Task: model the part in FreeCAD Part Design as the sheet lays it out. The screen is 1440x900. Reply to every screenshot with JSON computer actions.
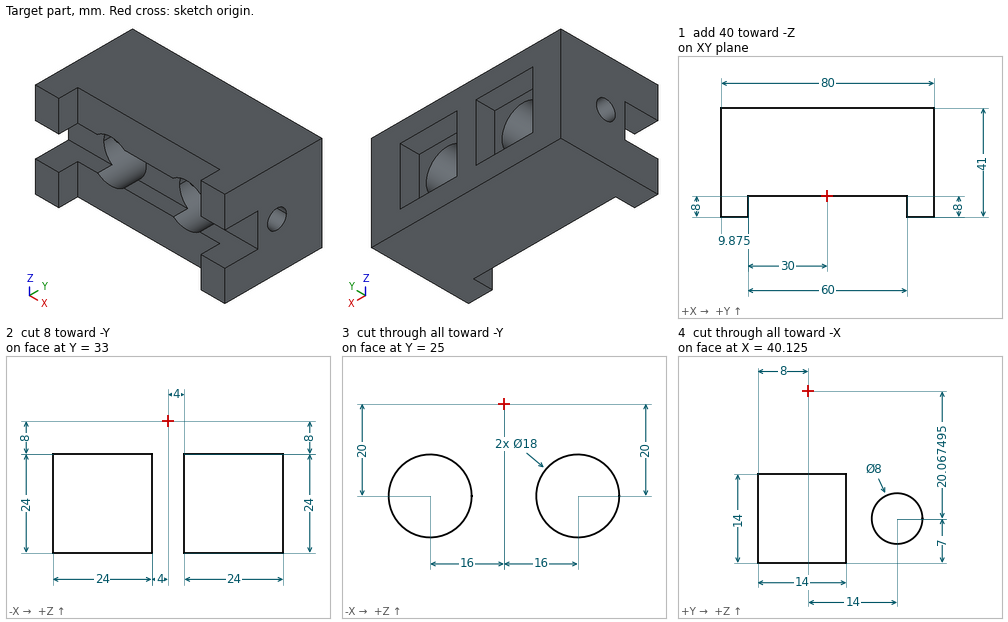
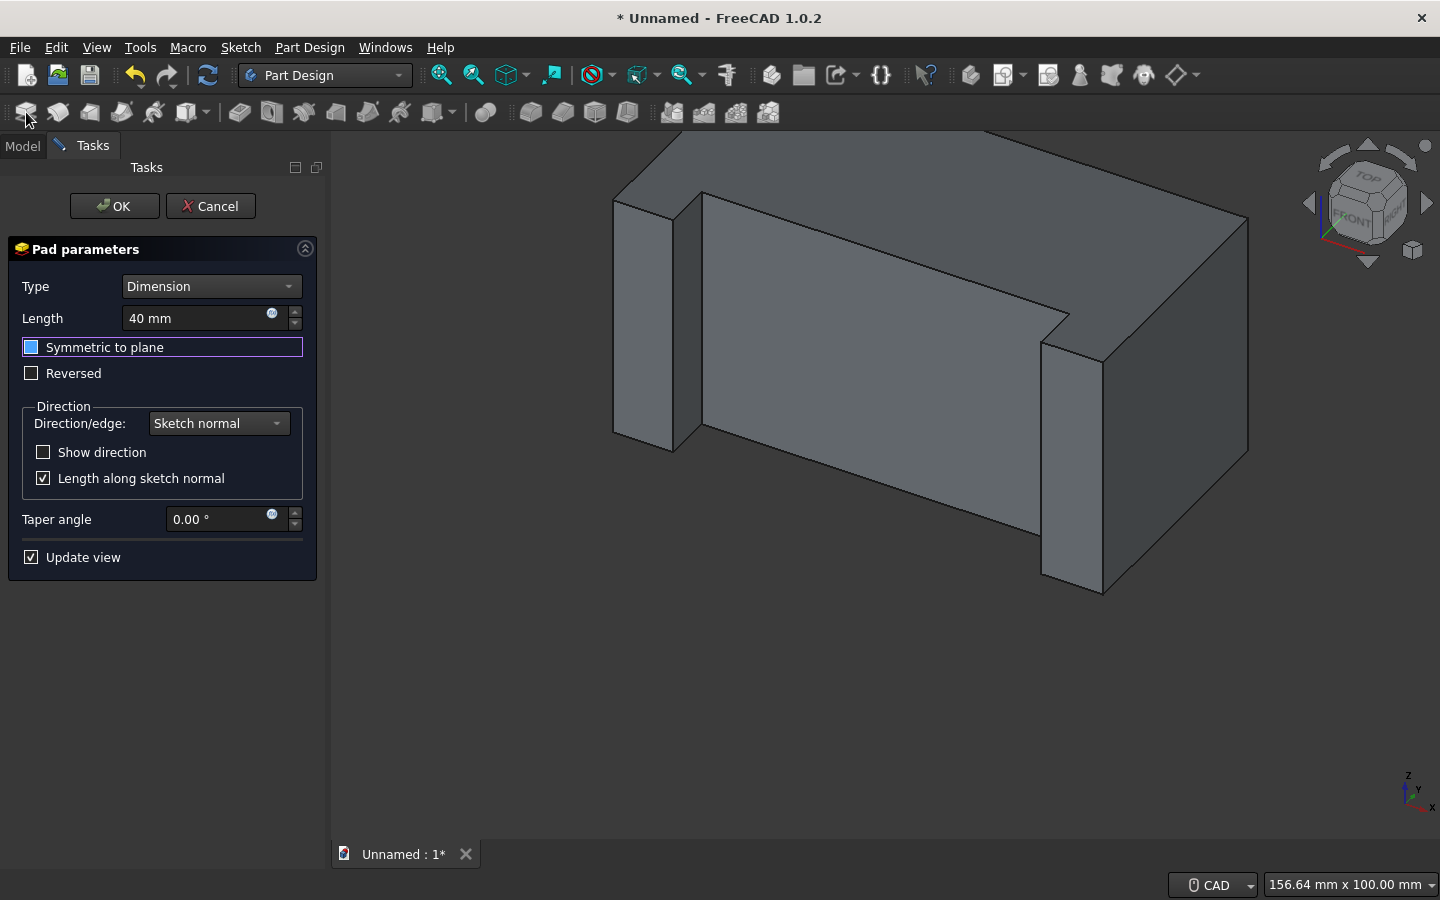
{"action": "left_click", "coordinate": [30, 373]}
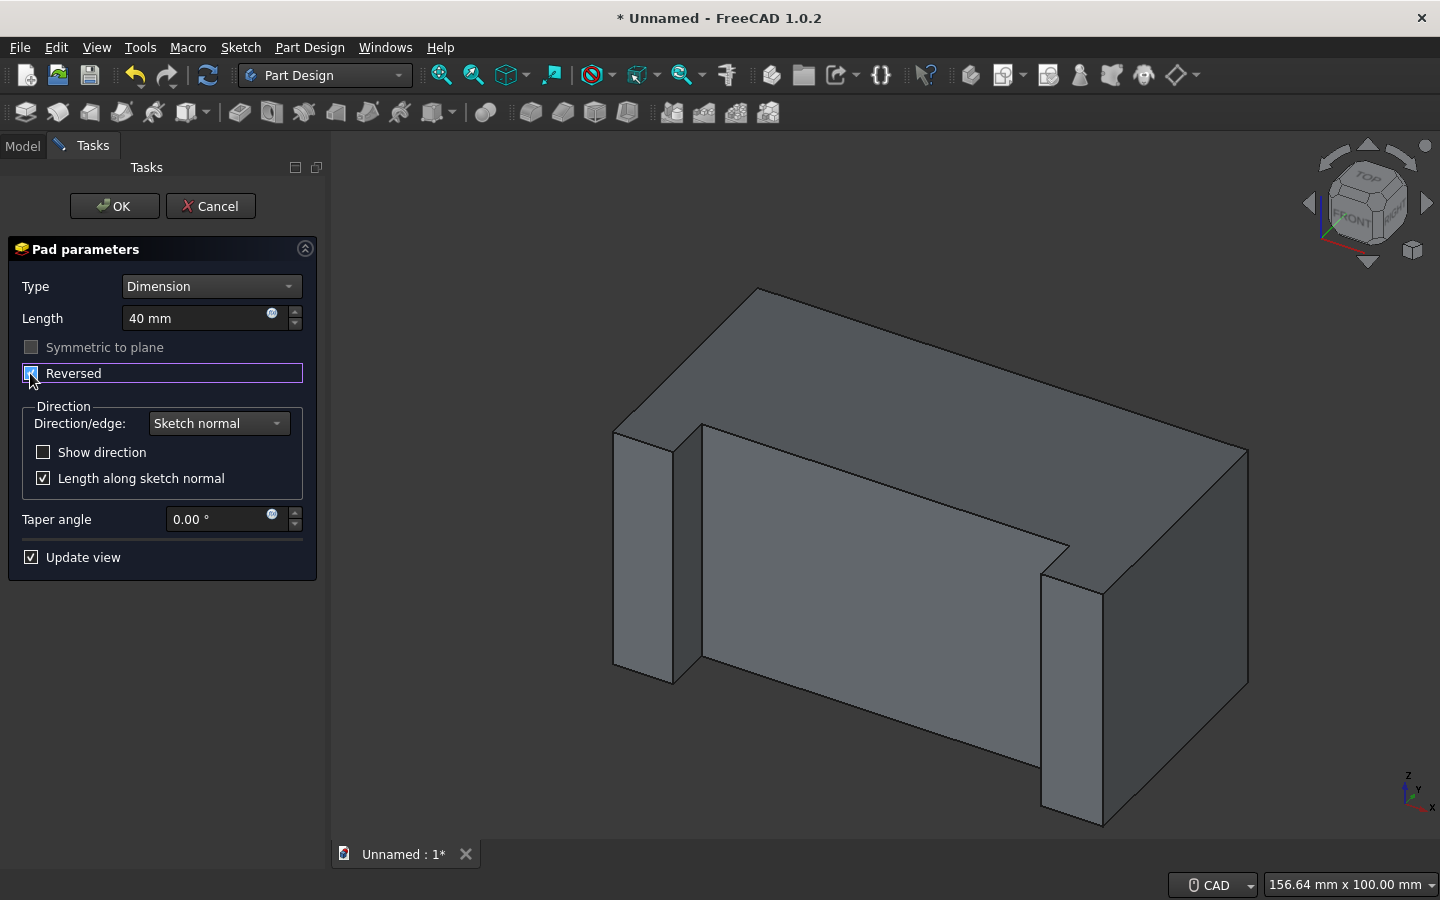
{"action": "left_click", "coordinate": [115, 206]}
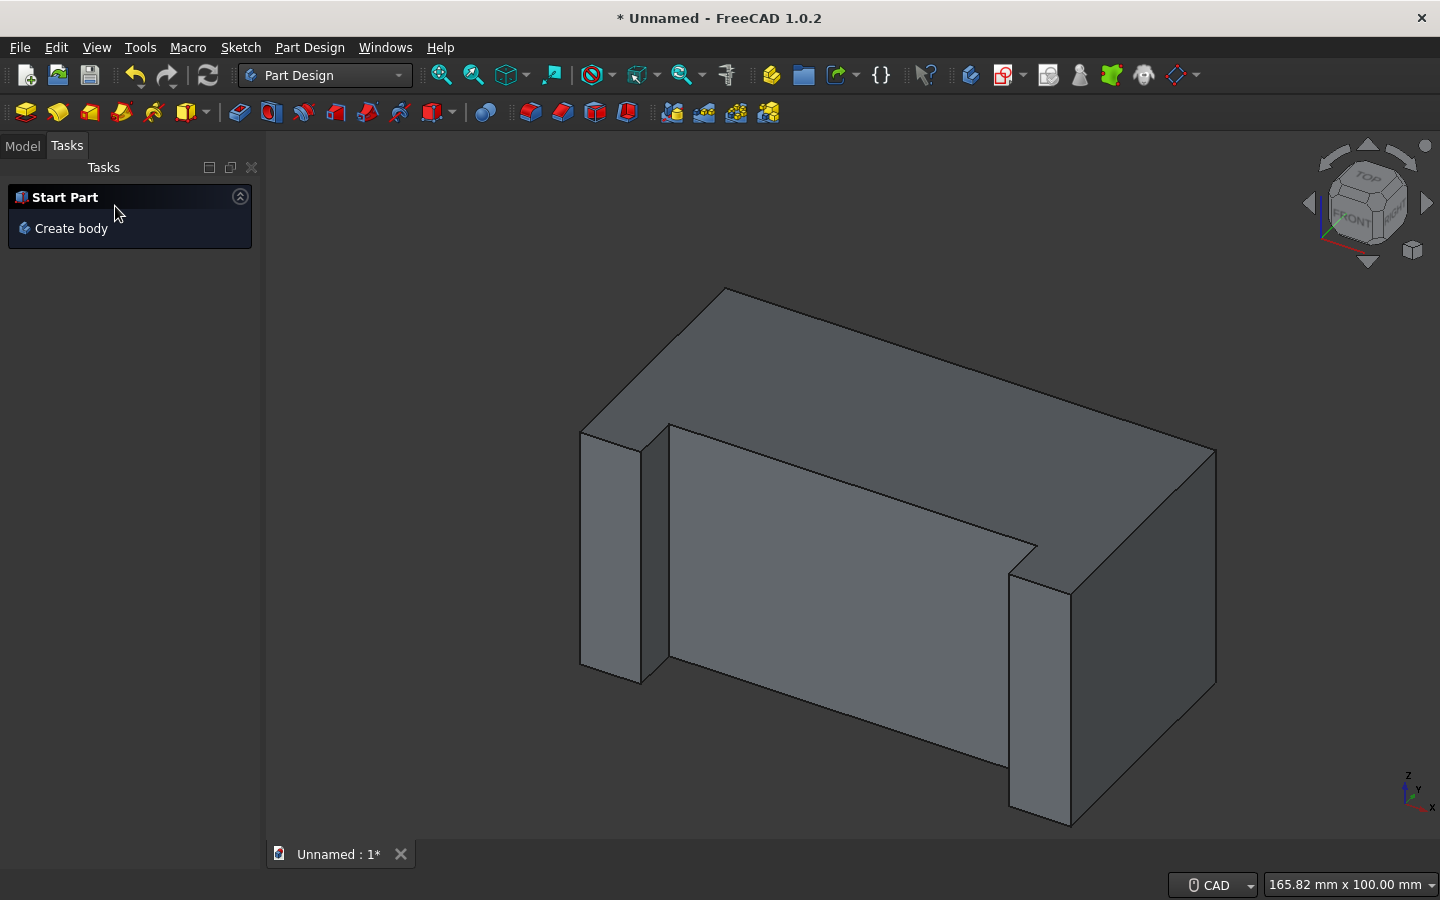
{"action": "key", "text": "4"}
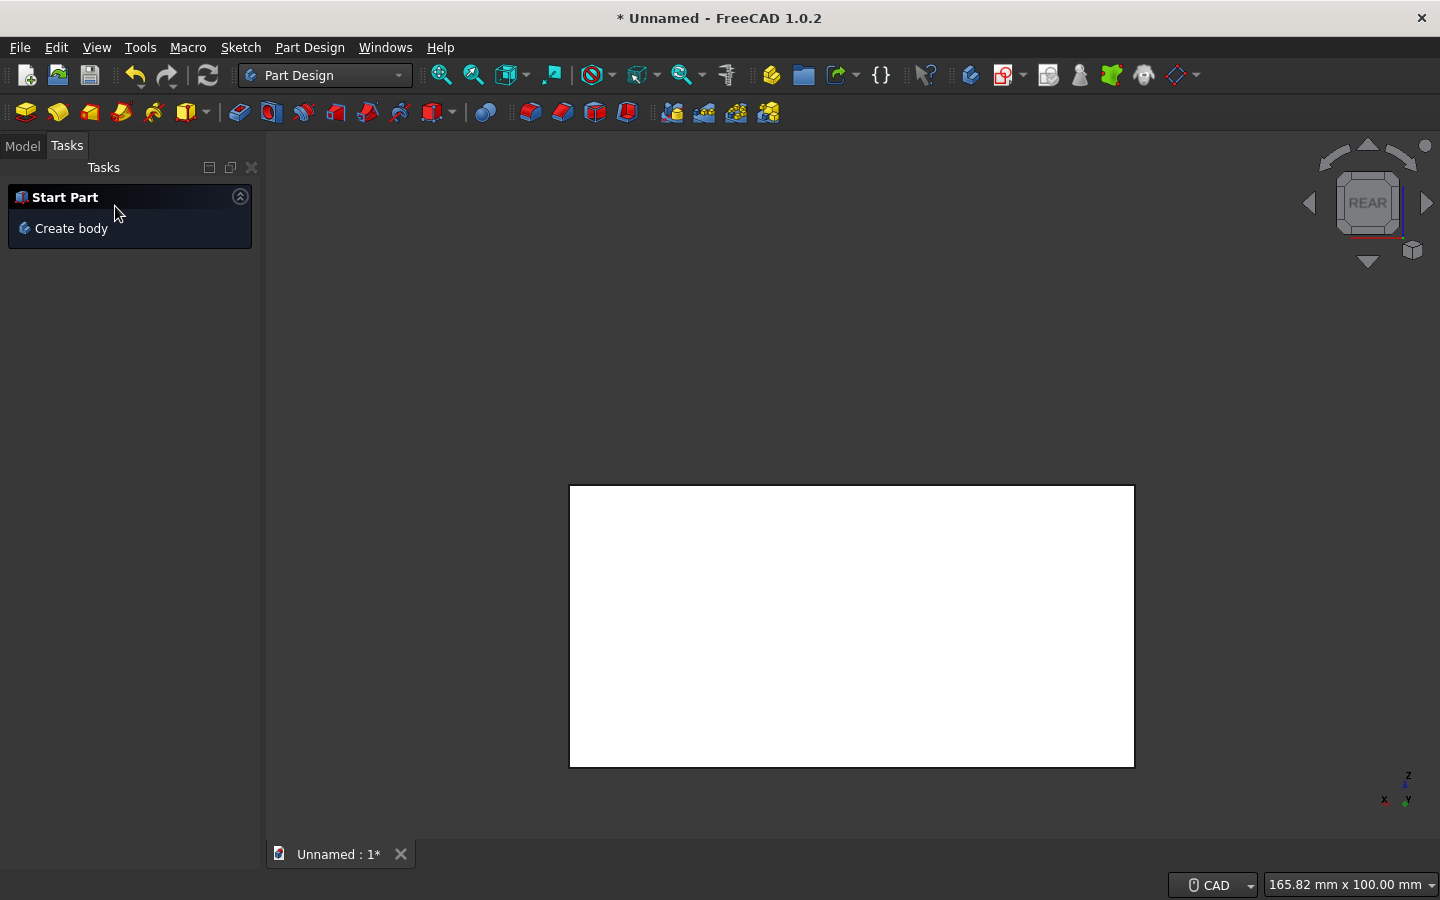
{"action": "left_click", "coordinate": [771, 626]}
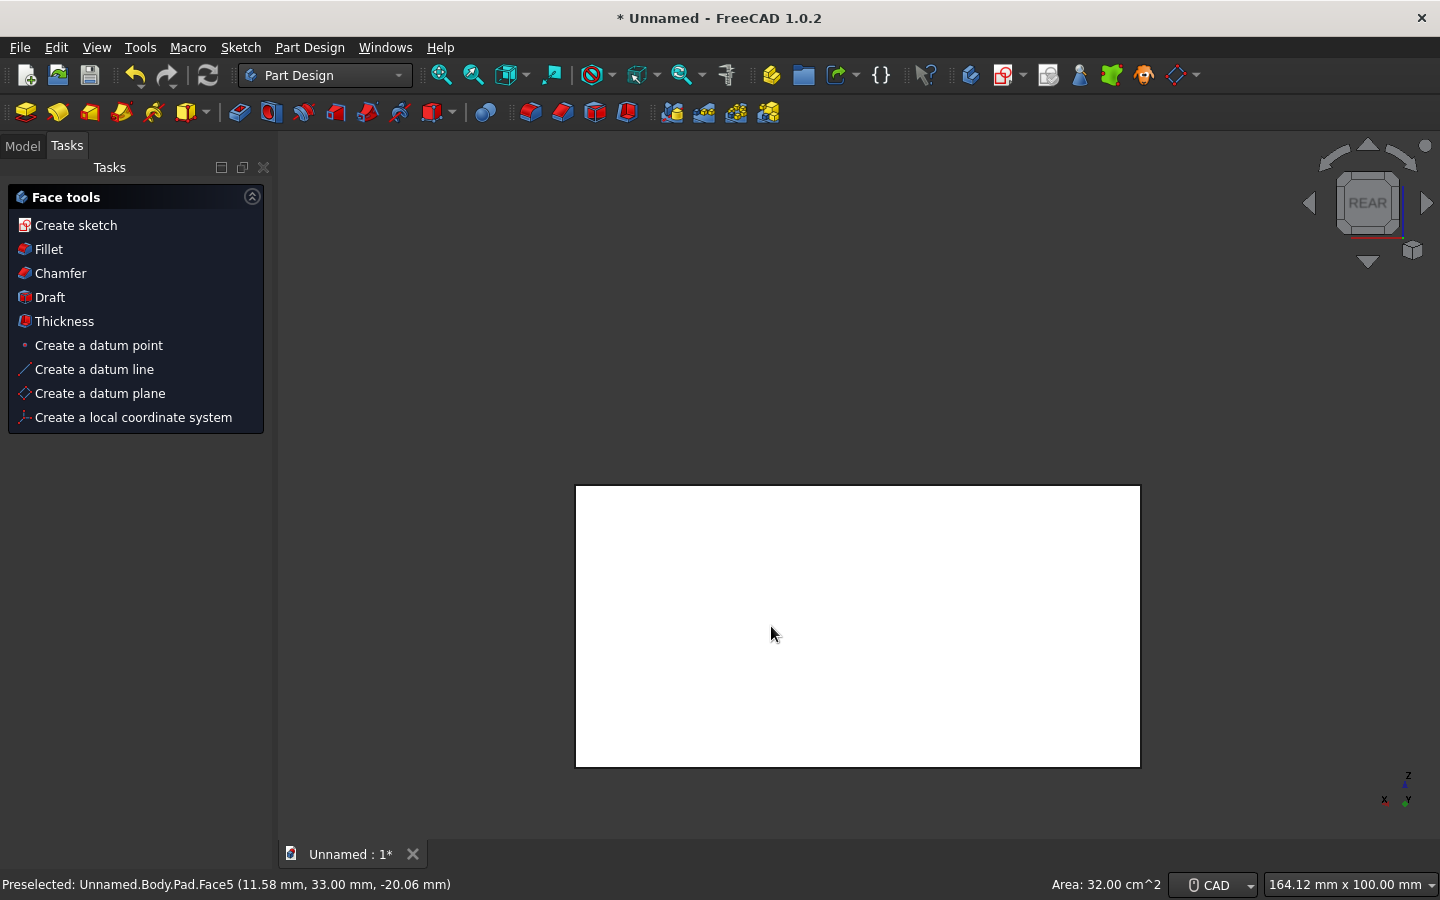
{"action": "left_click", "coordinate": [1004, 76]}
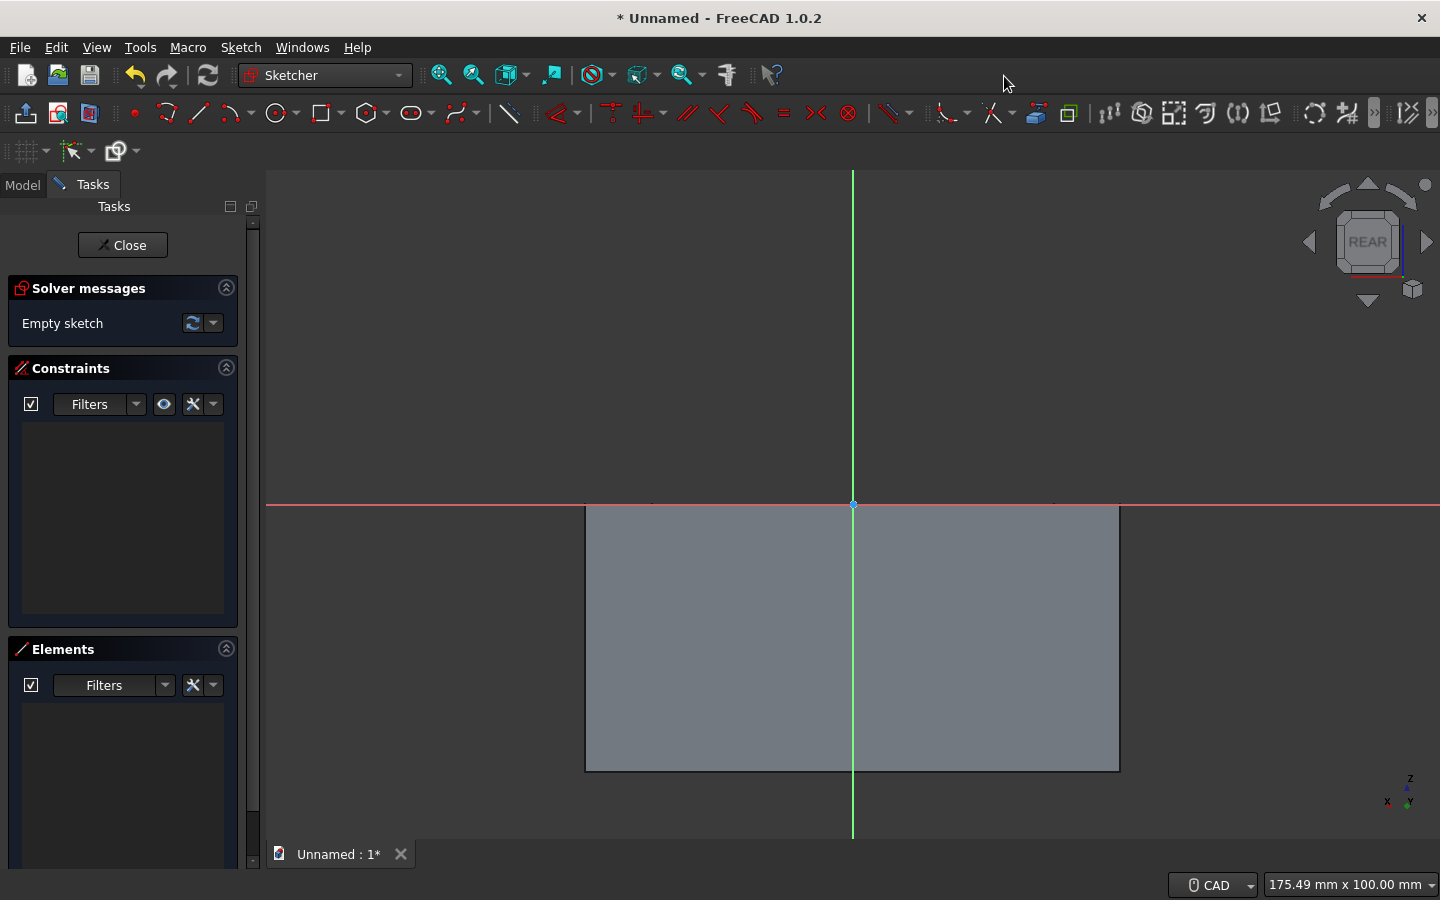
{"action": "scroll", "coordinate": [936, 742], "scroll_direction": "up", "scroll_amount": 3}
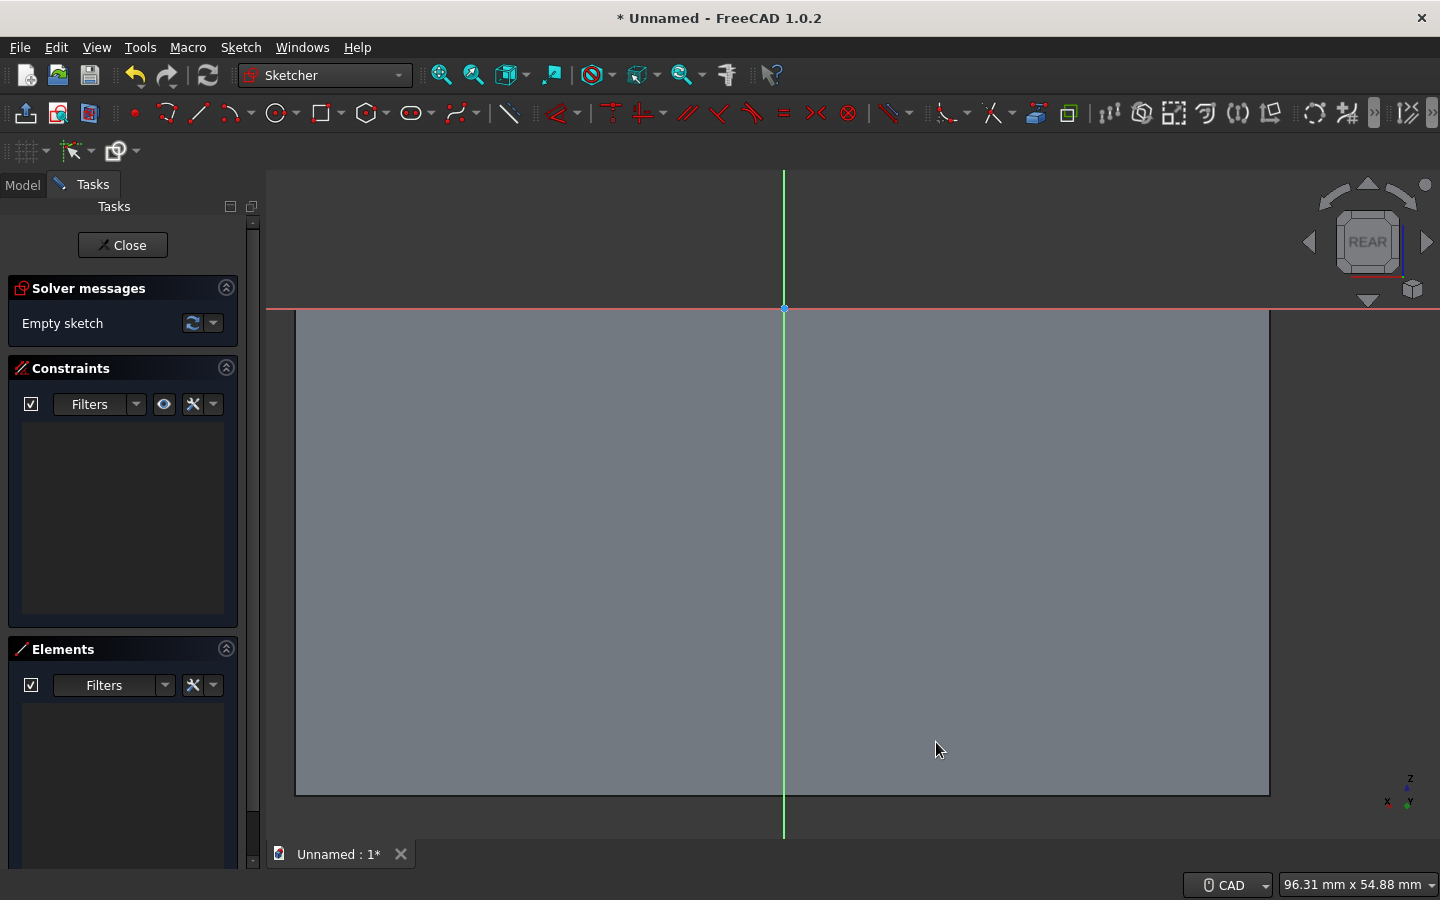
{"action": "key", "text": "g r"}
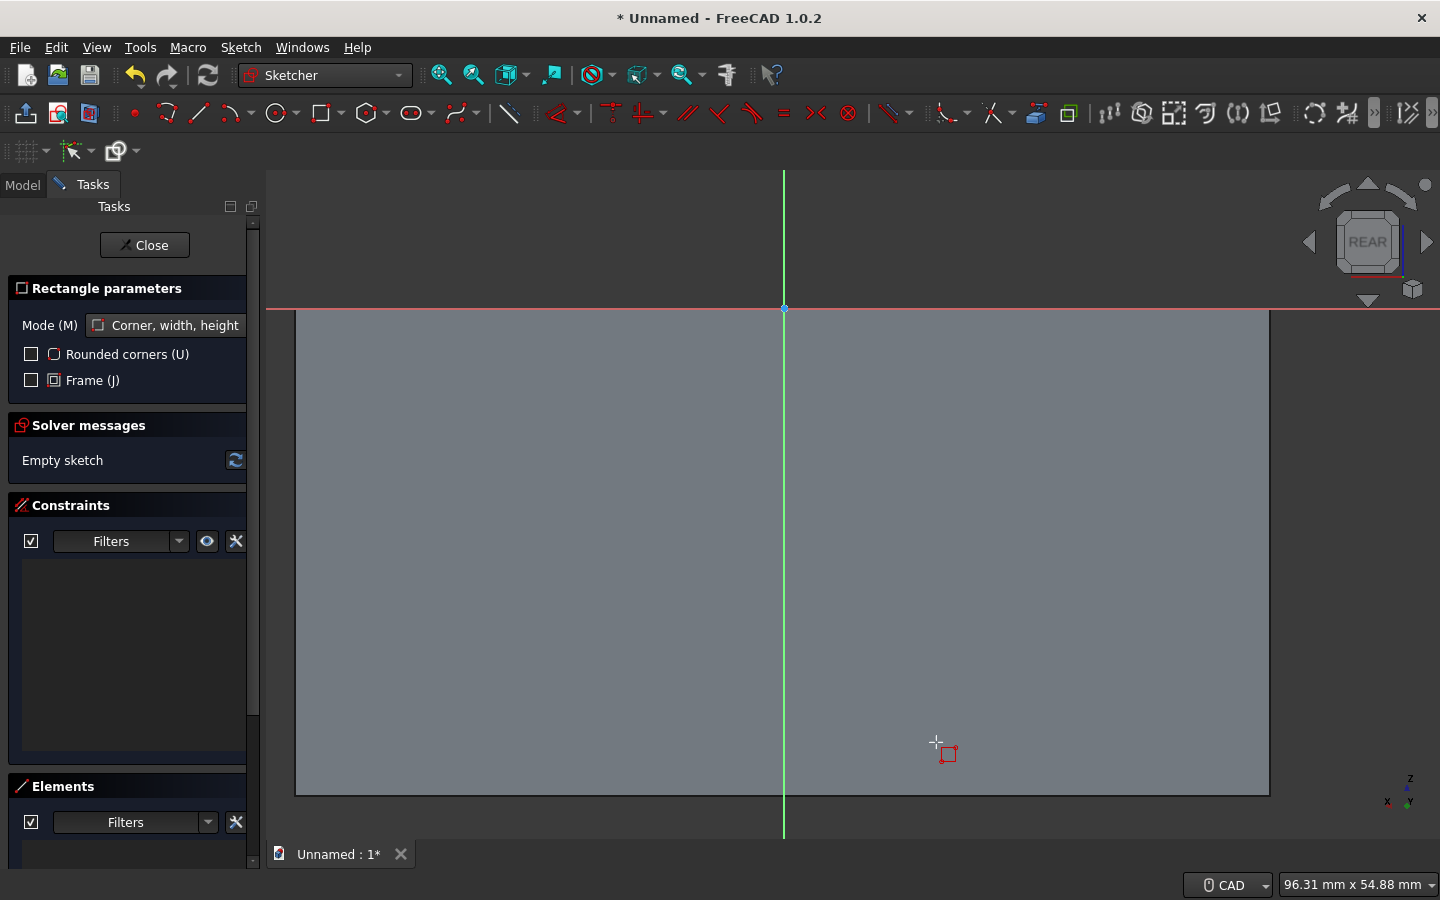
{"action": "left_click", "coordinate": [833, 406]}
{"action": "left_click", "coordinate": [1126, 699]}